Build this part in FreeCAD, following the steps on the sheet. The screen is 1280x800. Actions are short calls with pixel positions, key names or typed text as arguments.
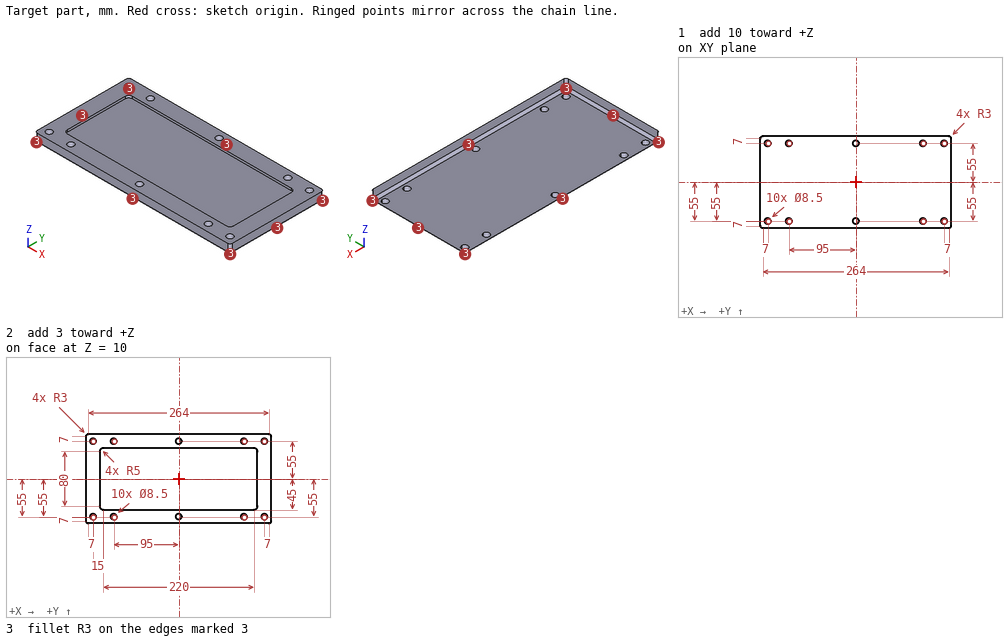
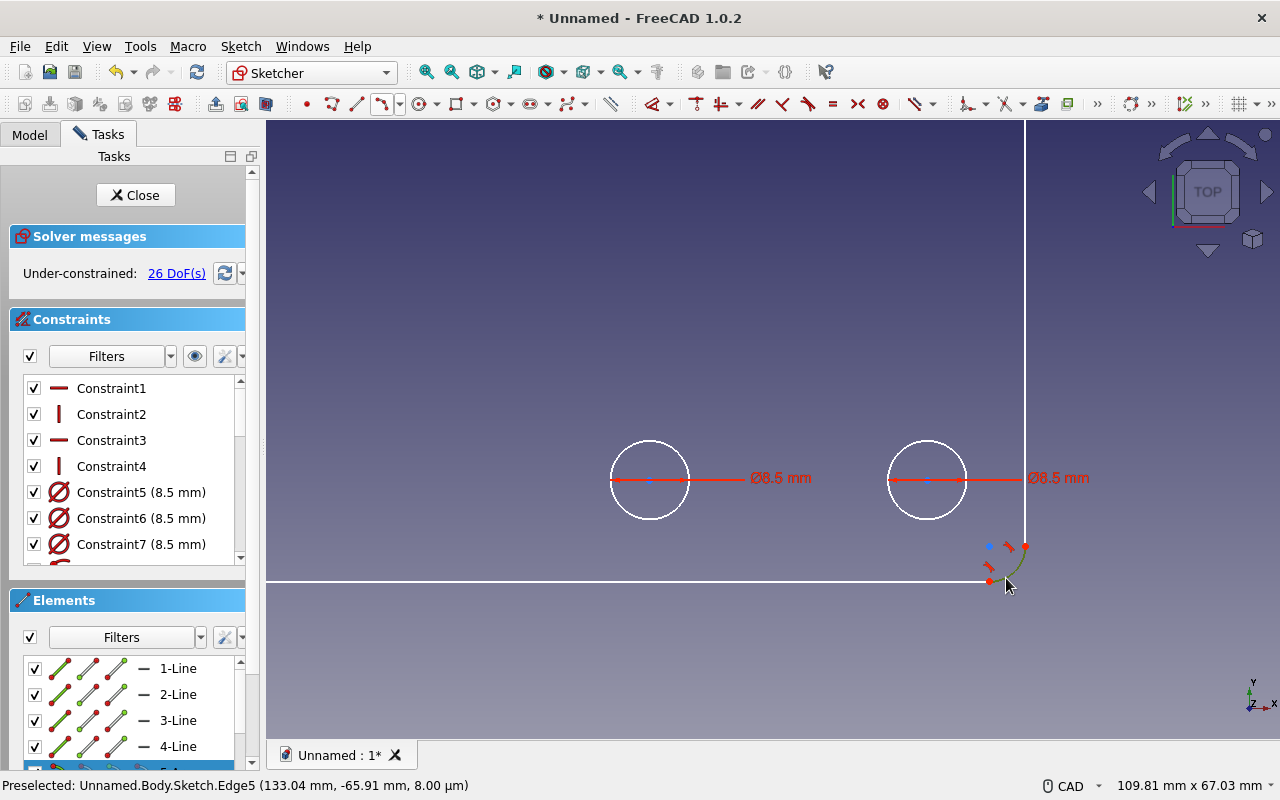
scroll(1009, 580, down, 7)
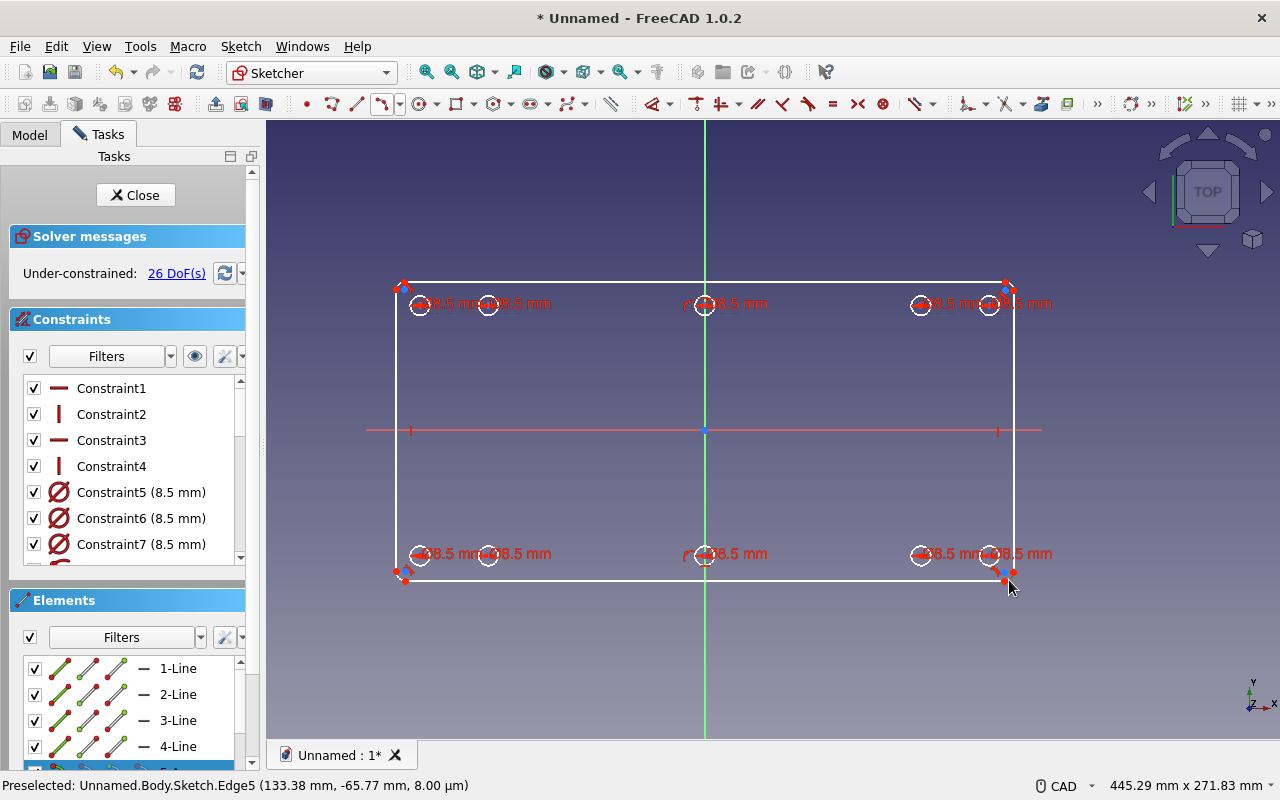
scroll(1013, 286, up, 7)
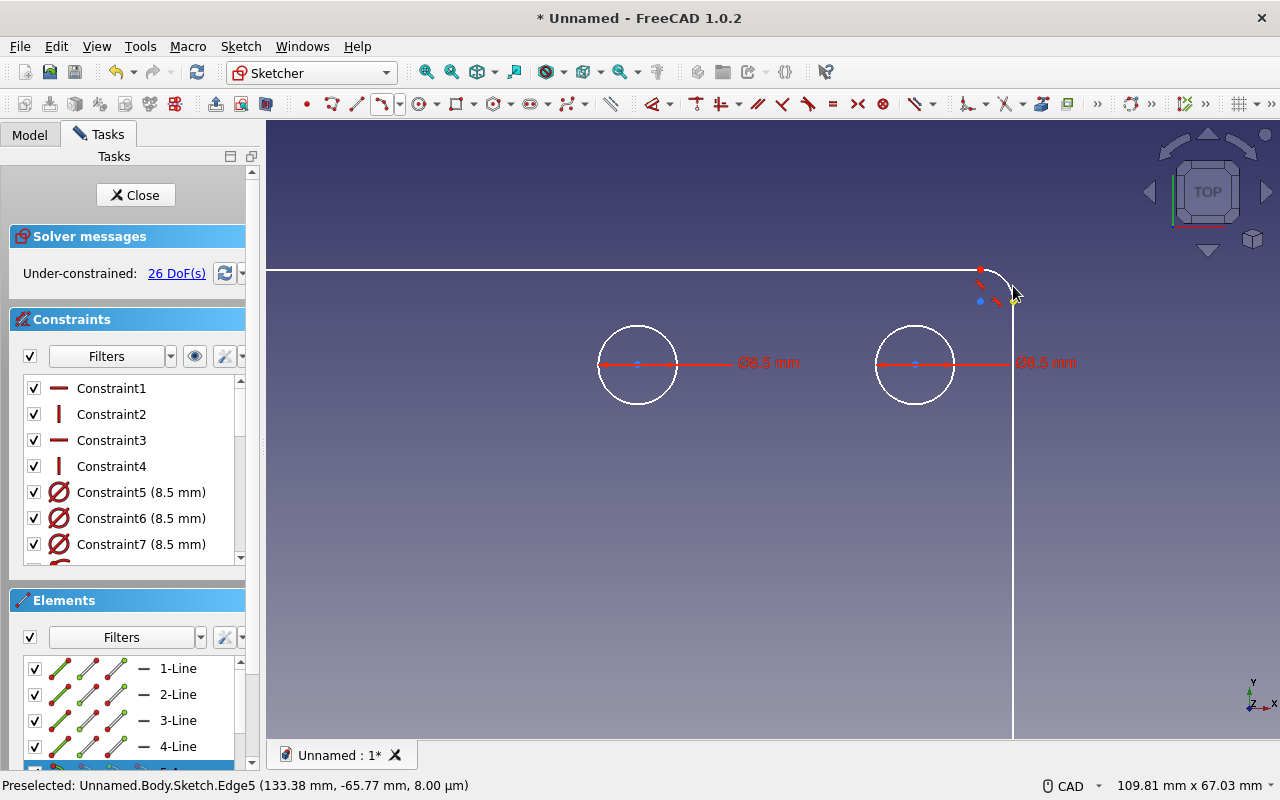
click(1010, 287)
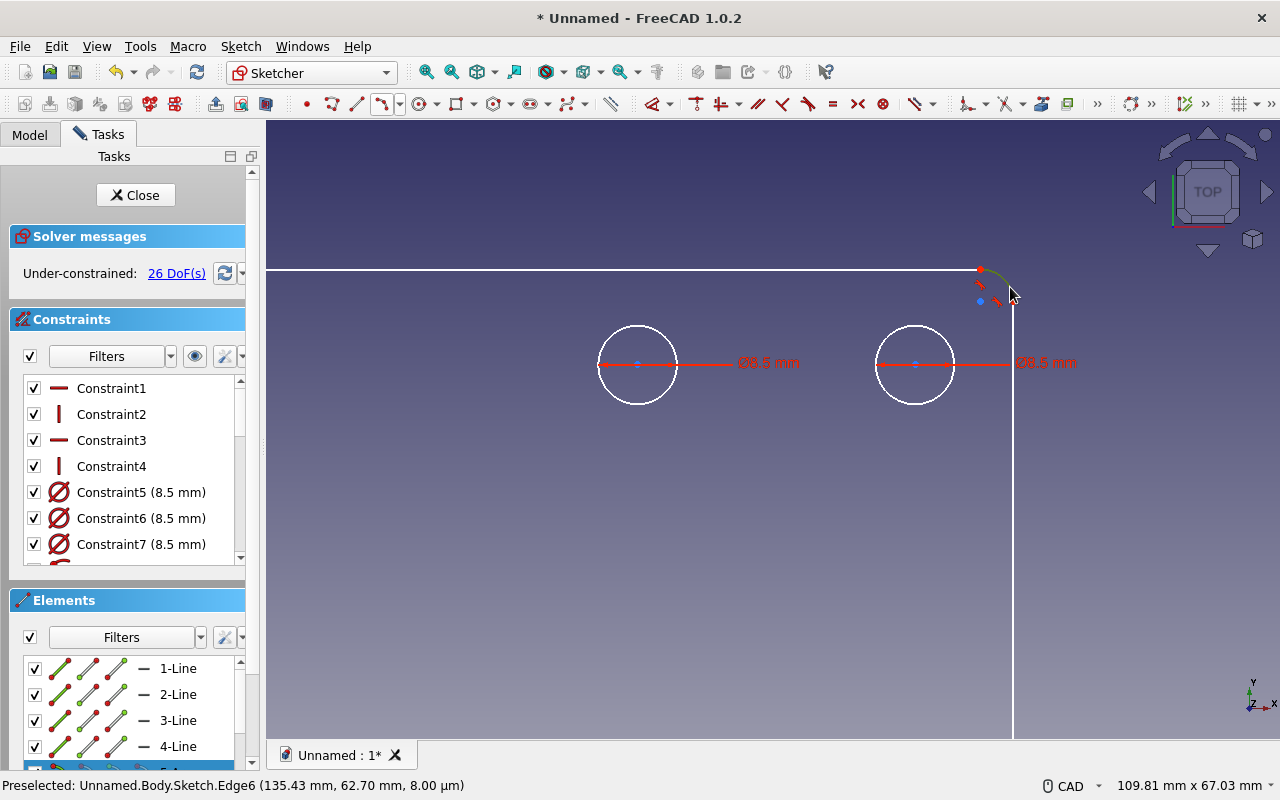
scroll(1013, 285, down, 7)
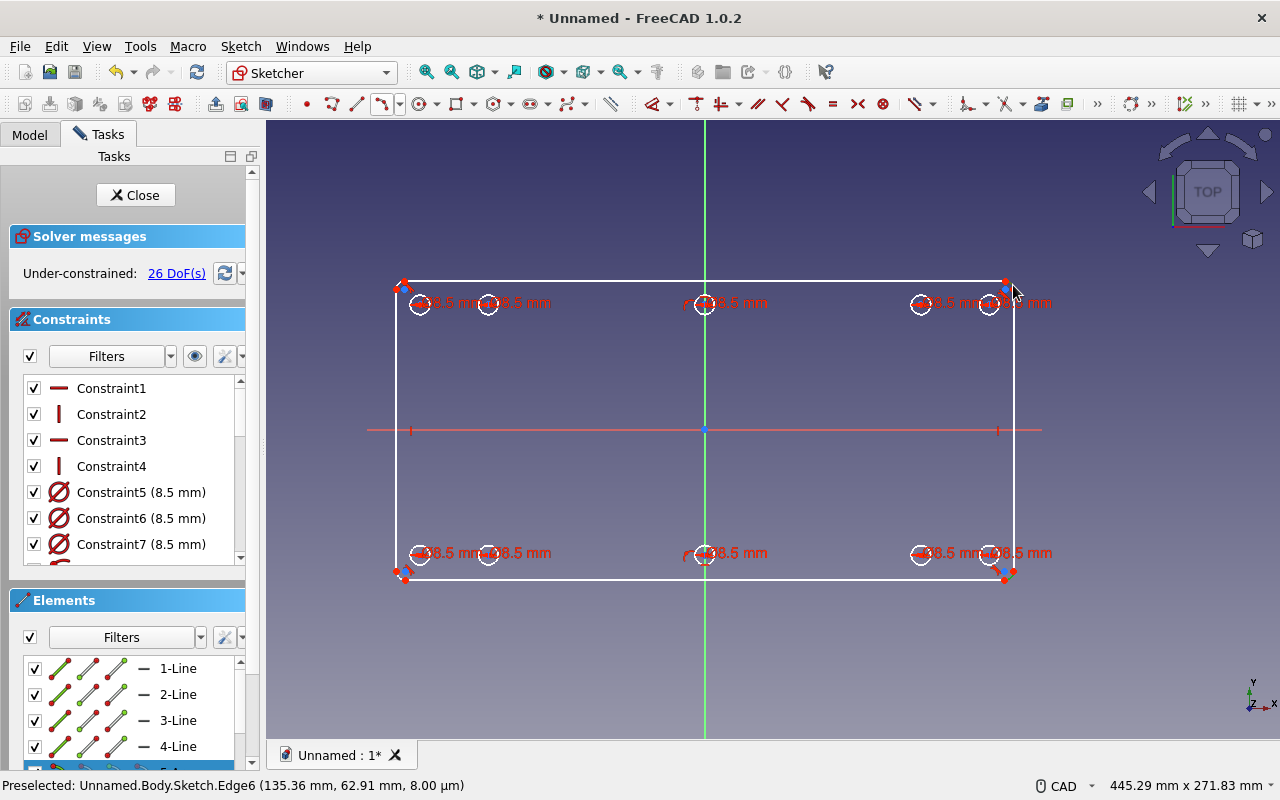
scroll(401, 282, up, 7)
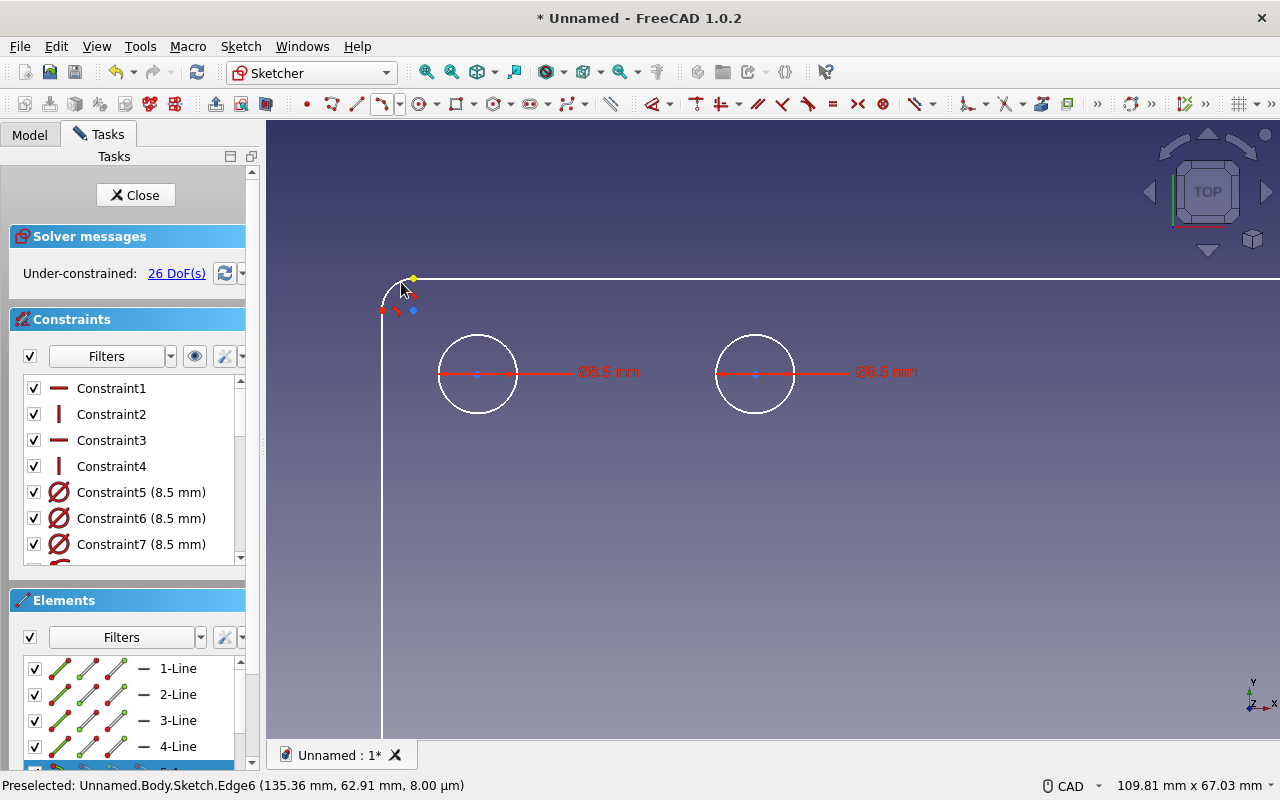
click(399, 282)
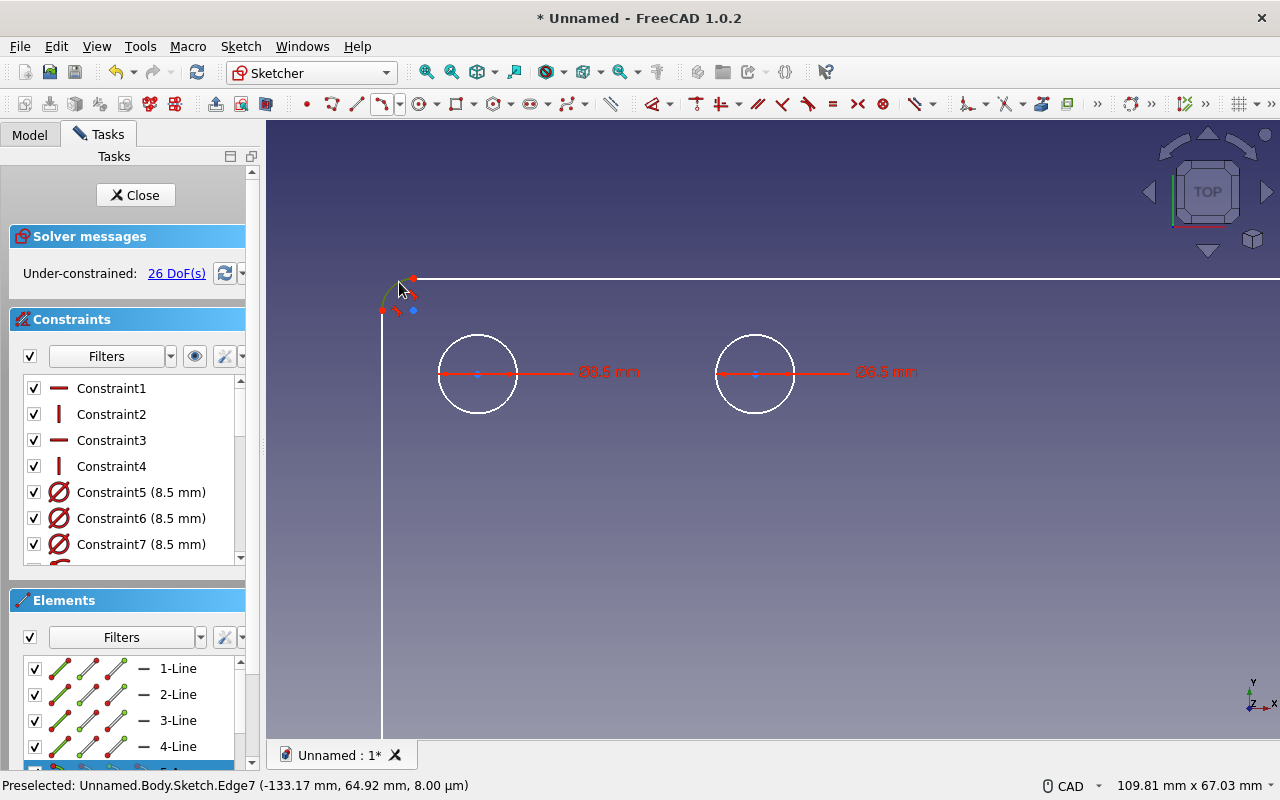
scroll(401, 282, down, 7)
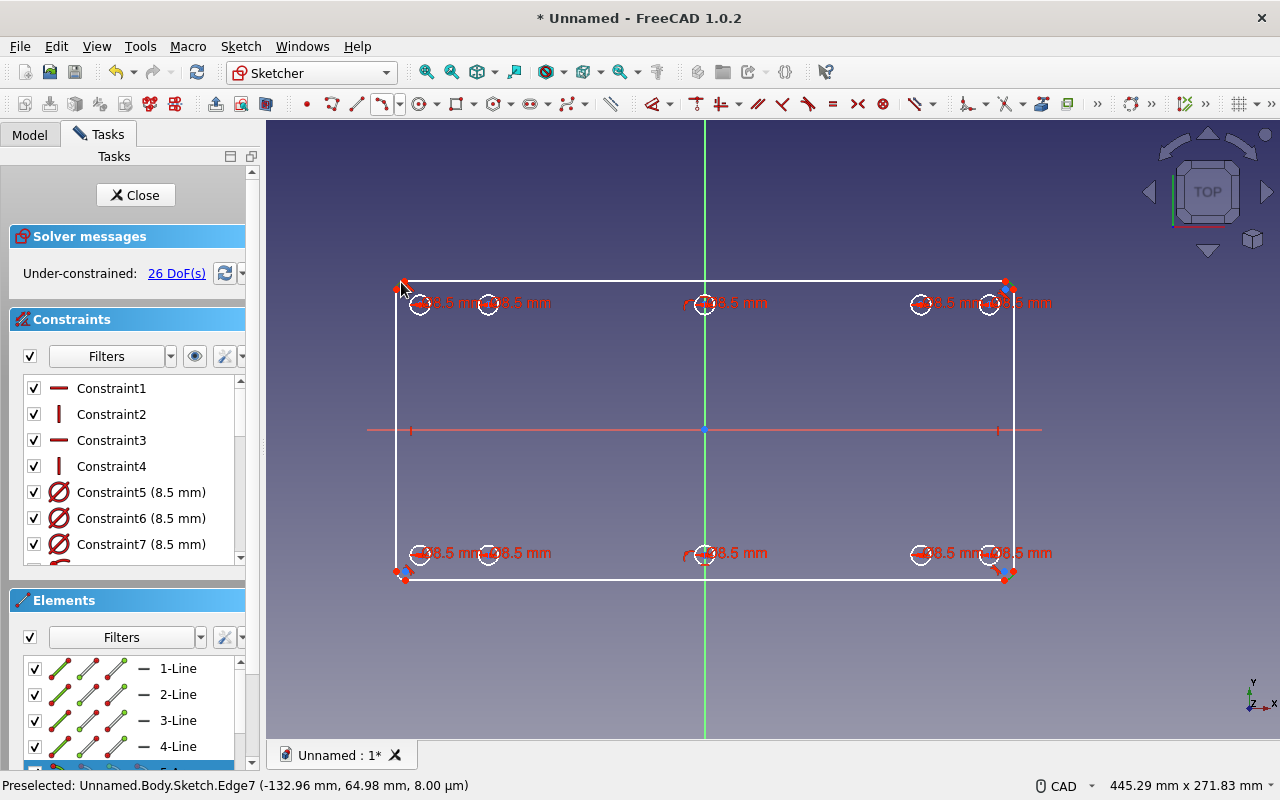
scroll(397, 575, up, 6)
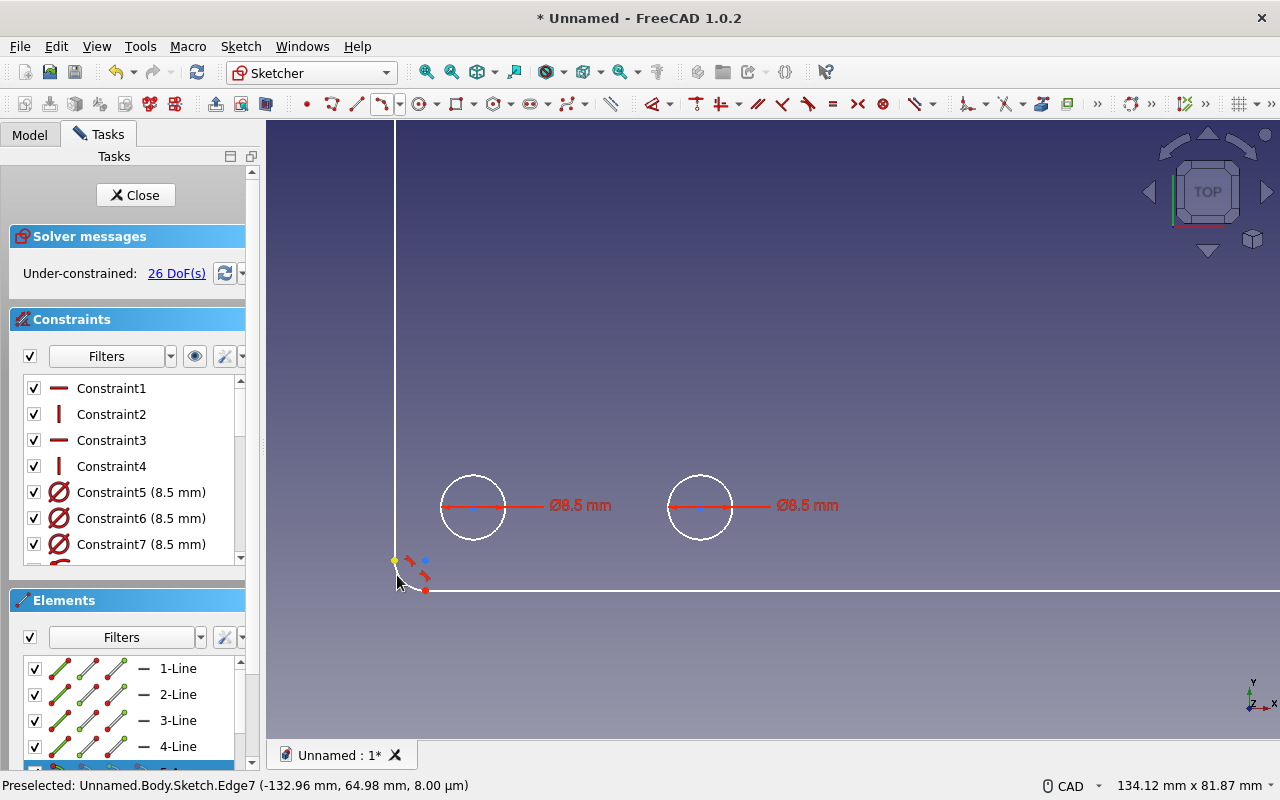
click(398, 574)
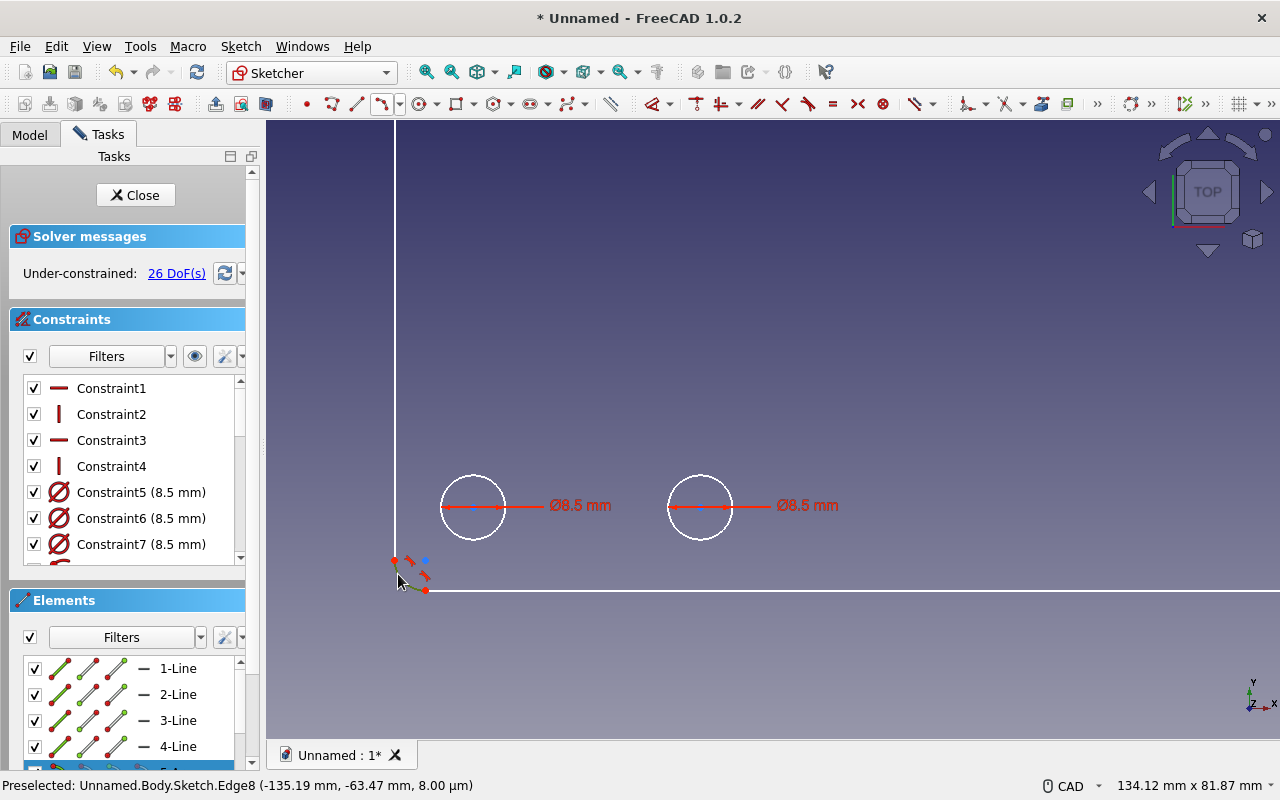
click(833, 104)